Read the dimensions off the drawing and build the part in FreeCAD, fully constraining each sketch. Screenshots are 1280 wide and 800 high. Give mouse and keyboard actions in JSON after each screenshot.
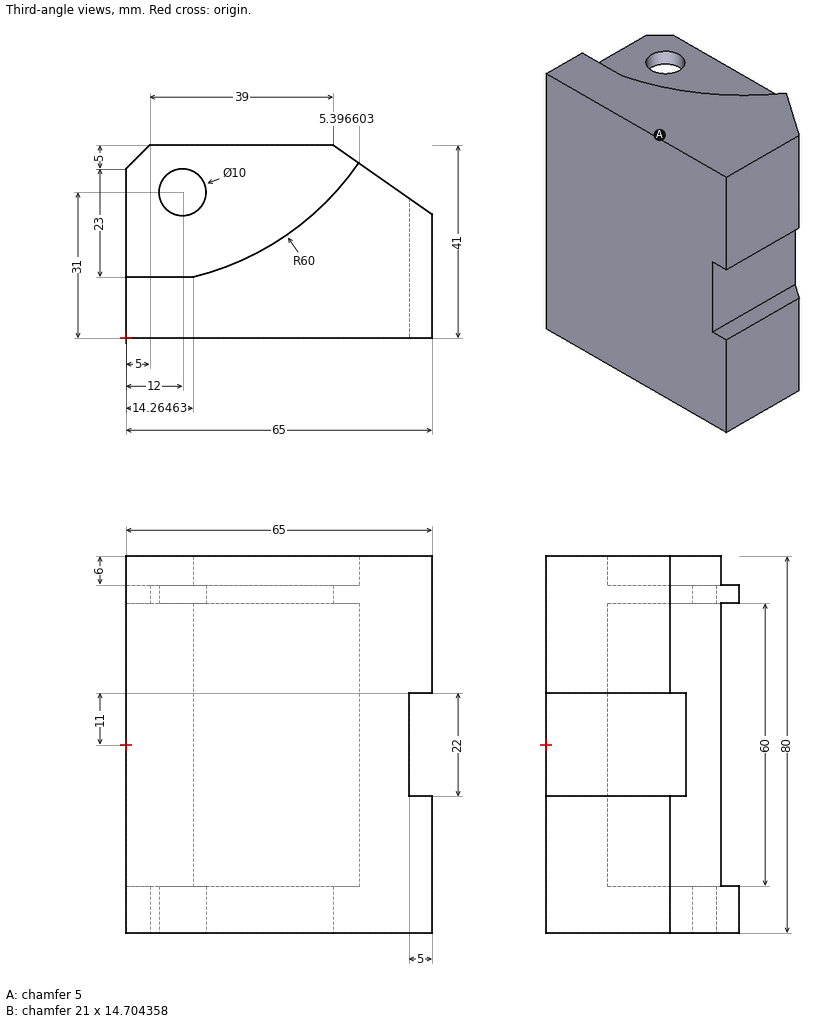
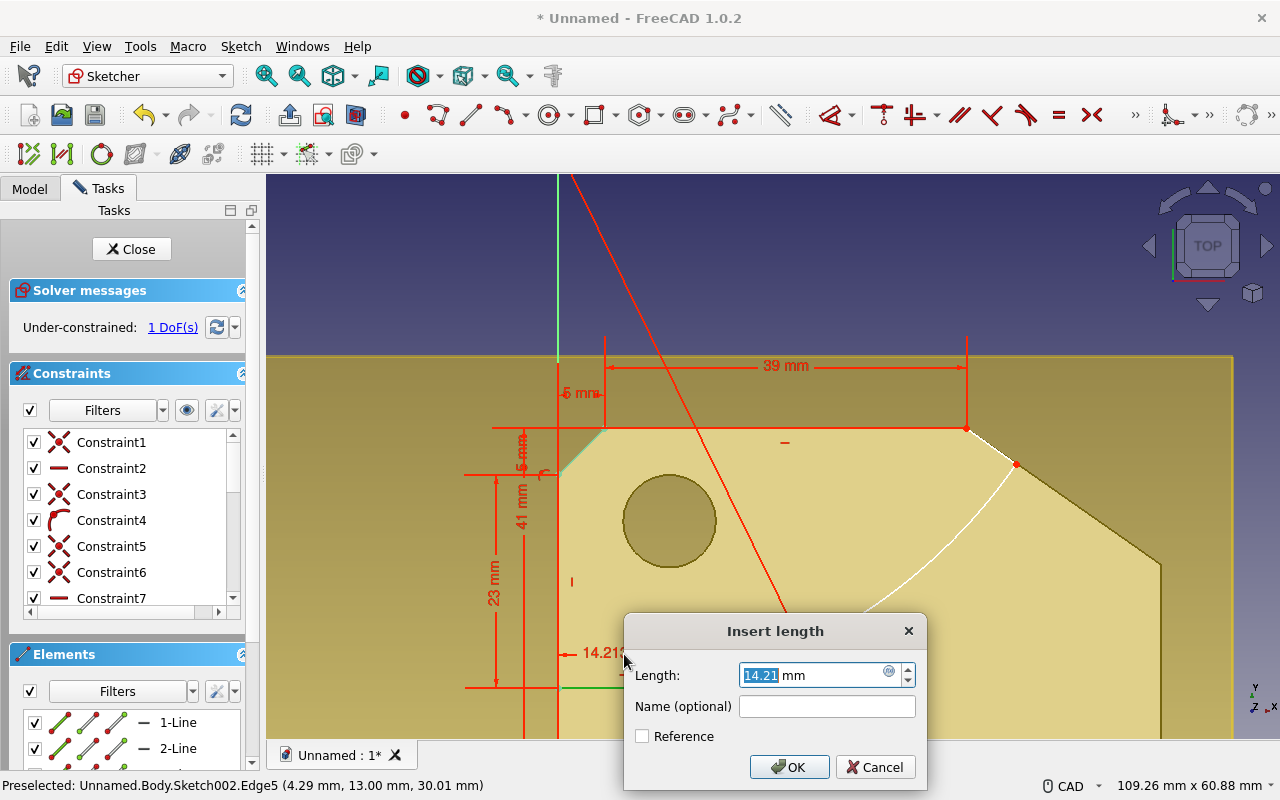
{"action": "type", "text": "14.26463"}
{"action": "key", "text": "Return"}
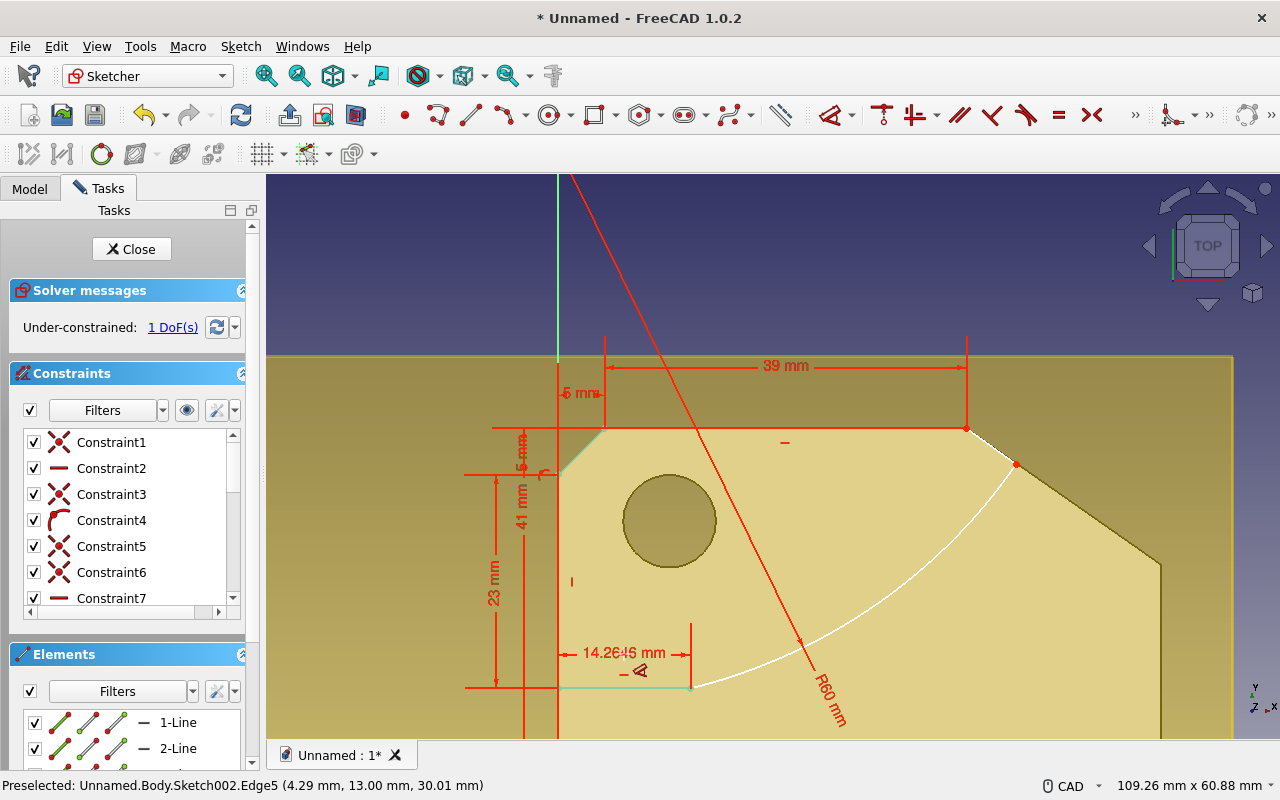
{"action": "left_click", "coordinate": [1001, 454]}
{"action": "left_click", "coordinate": [991, 394]}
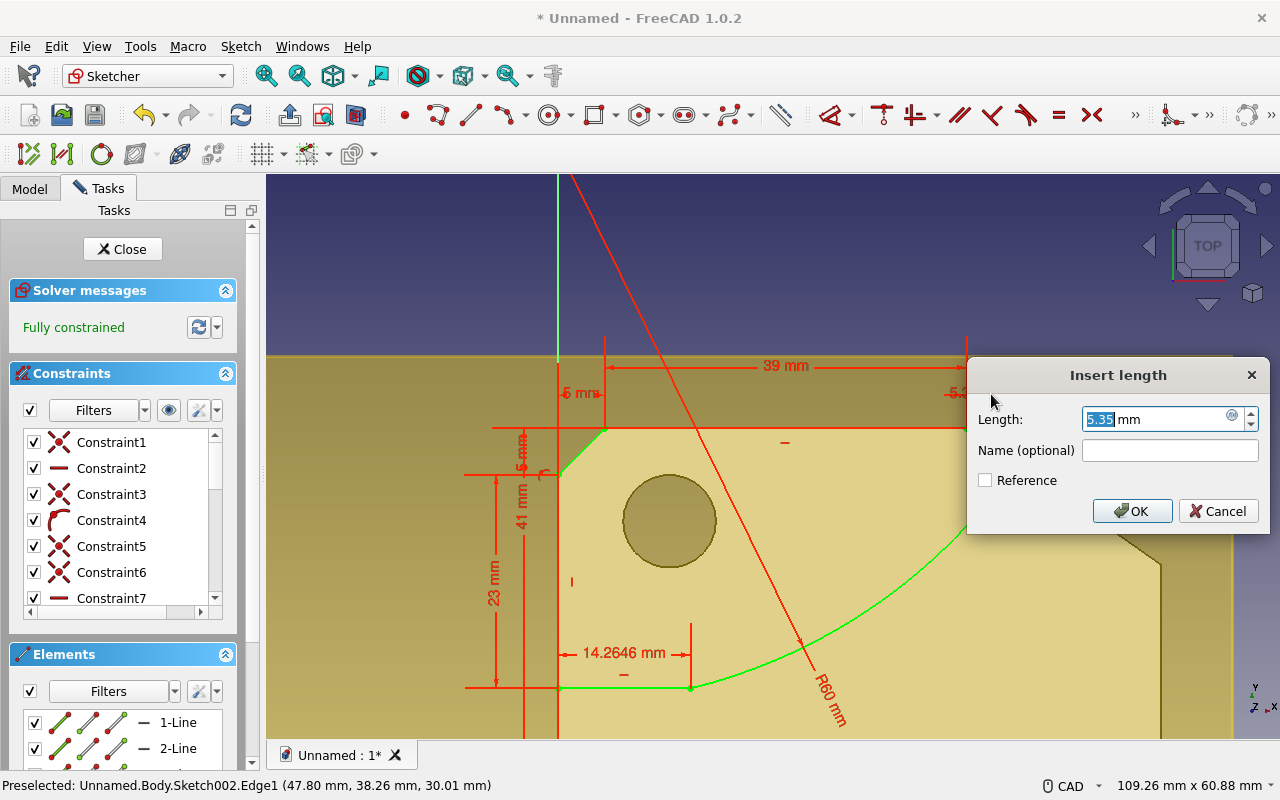
{"action": "type", "text": "5.396603"}
{"action": "key", "text": "Return"}
{"action": "key", "text": "Escape"}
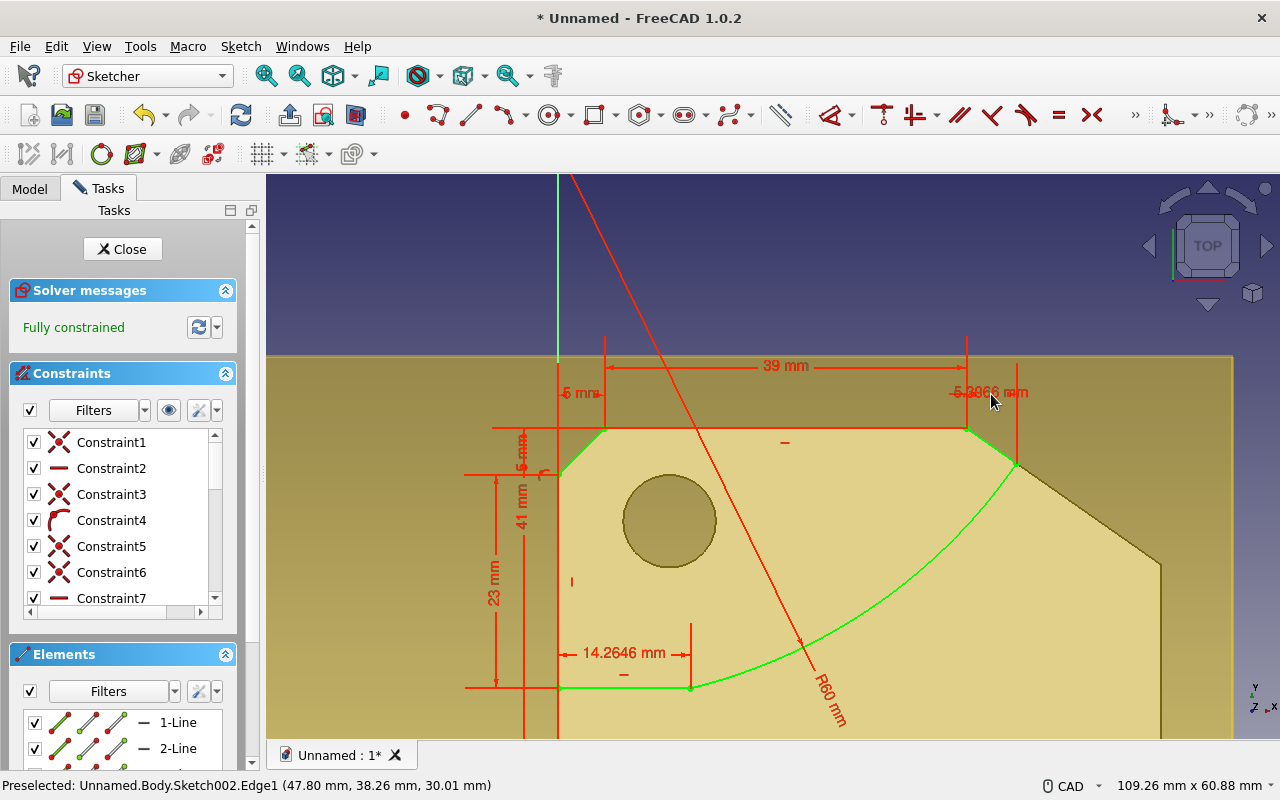
{"action": "left_click", "coordinate": [123, 249]}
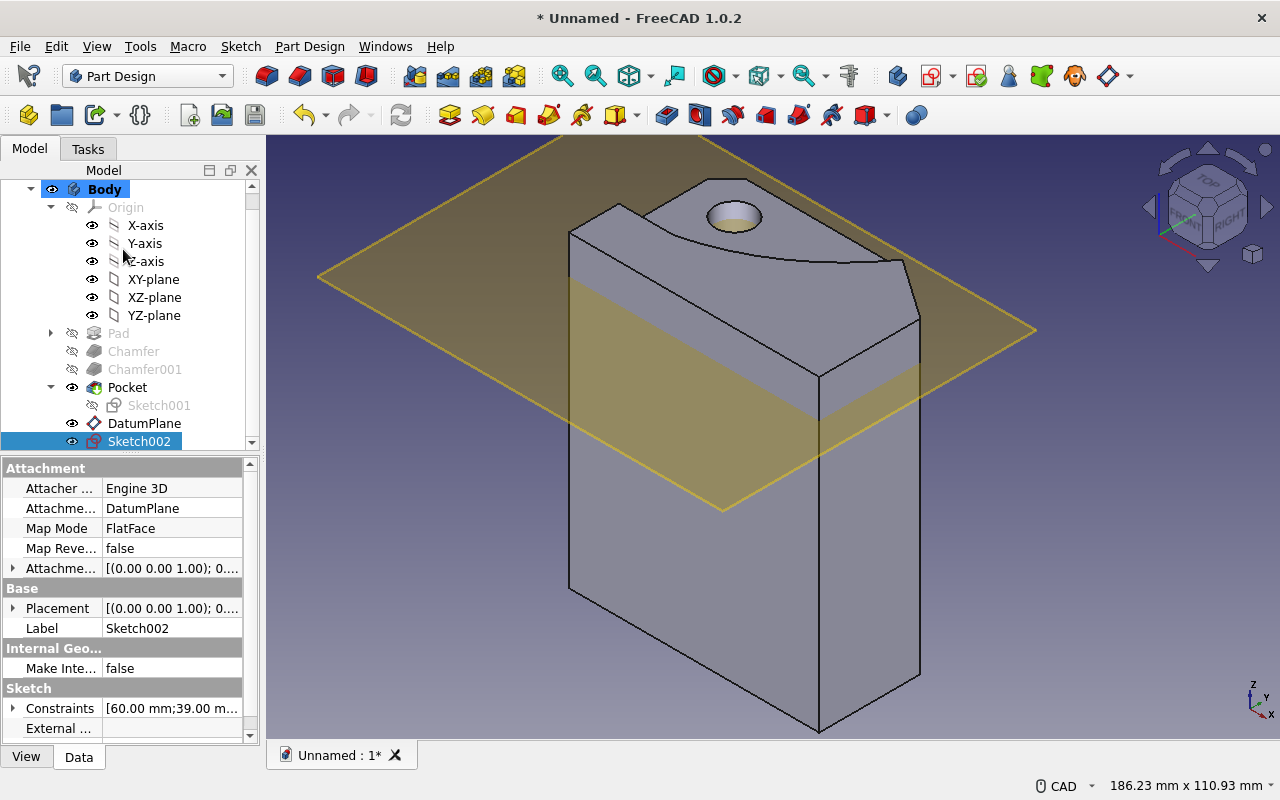
{"action": "left_click", "coordinate": [667, 116]}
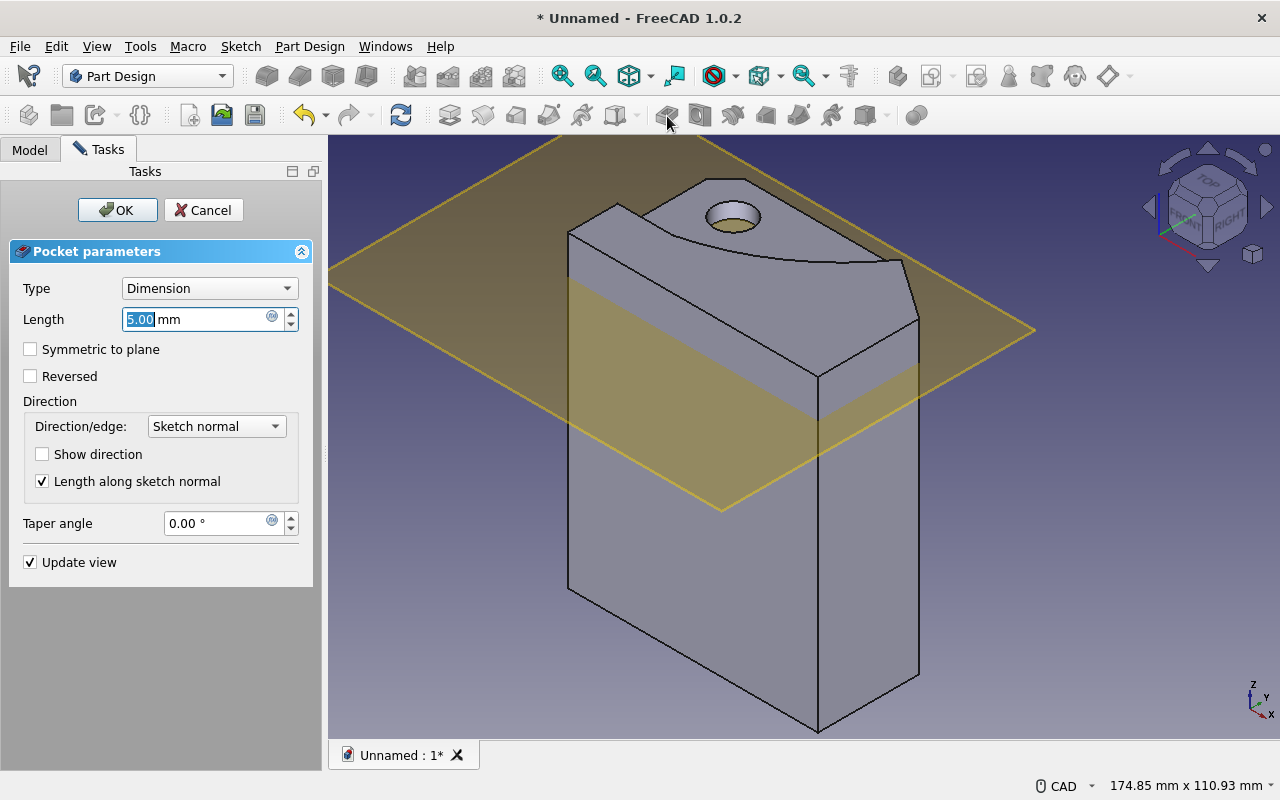
{"action": "type", "text": "60"}
{"action": "key", "text": "Tab"}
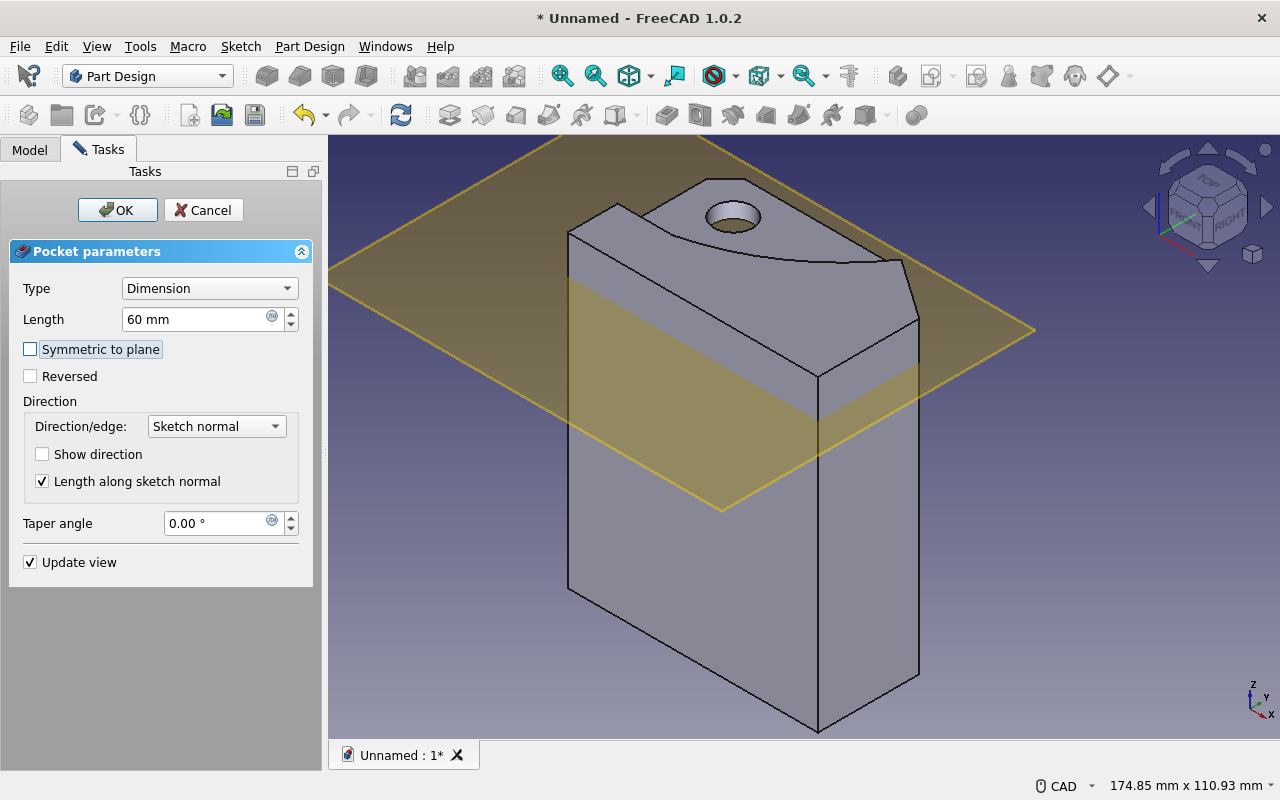
{"action": "left_click", "coordinate": [118, 210]}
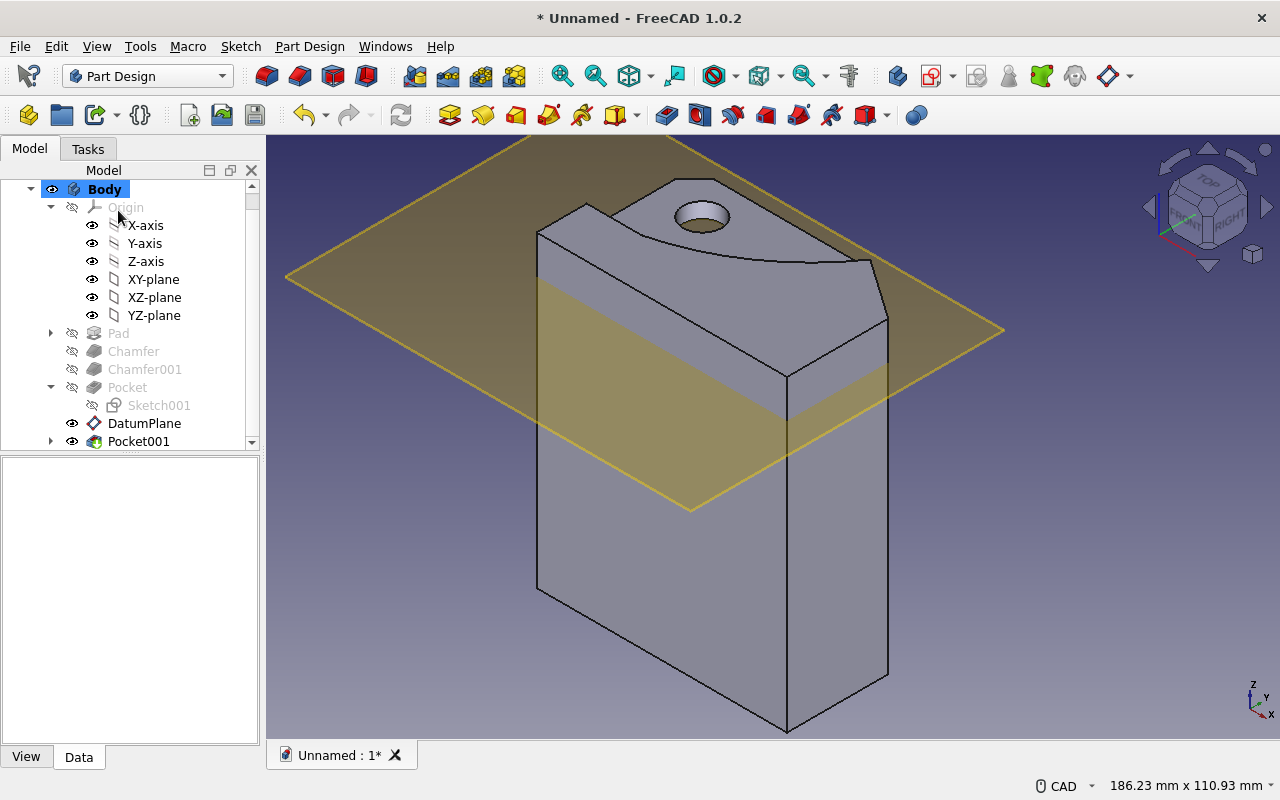
{"action": "left_click", "coordinate": [117, 423]}
{"action": "key", "text": "space"}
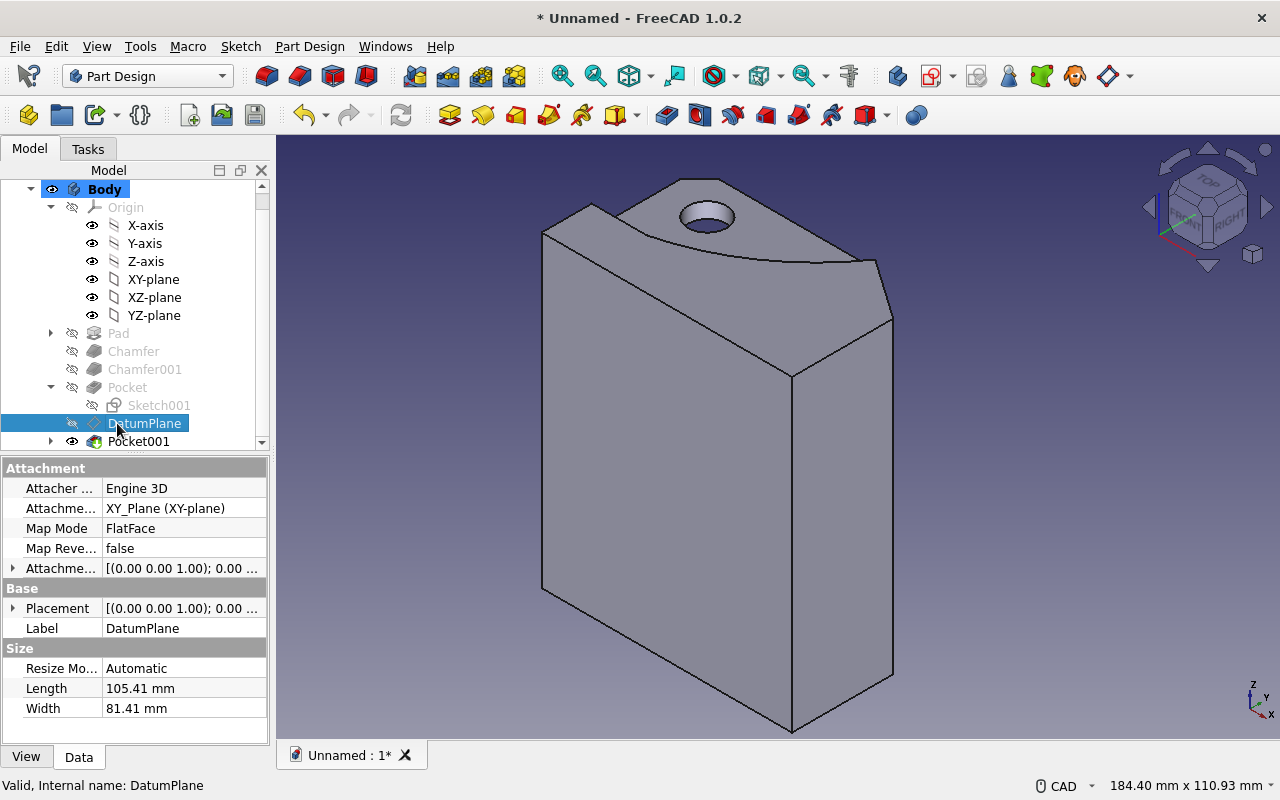
{"action": "key", "text": "4"}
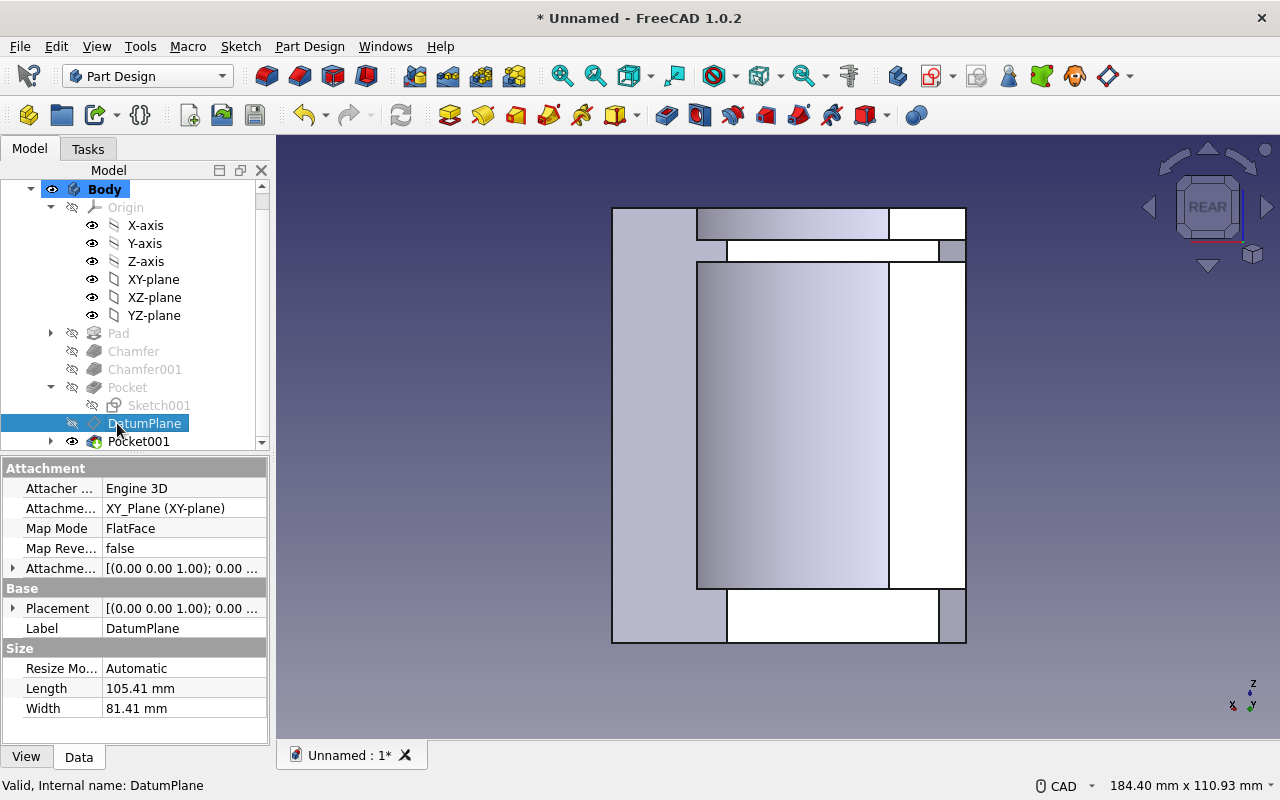
{"action": "left_click", "coordinate": [772, 615]}